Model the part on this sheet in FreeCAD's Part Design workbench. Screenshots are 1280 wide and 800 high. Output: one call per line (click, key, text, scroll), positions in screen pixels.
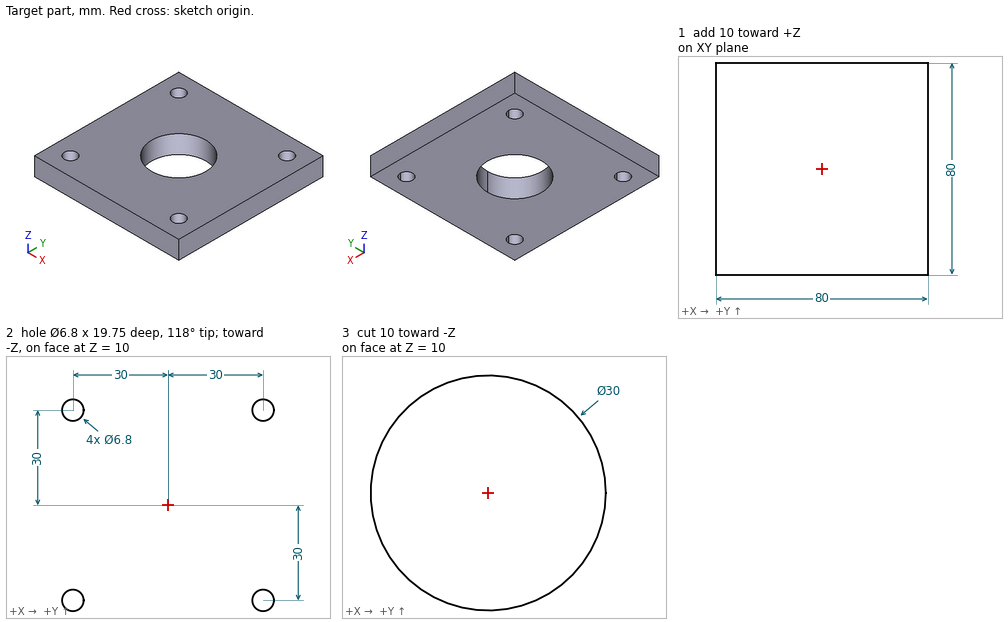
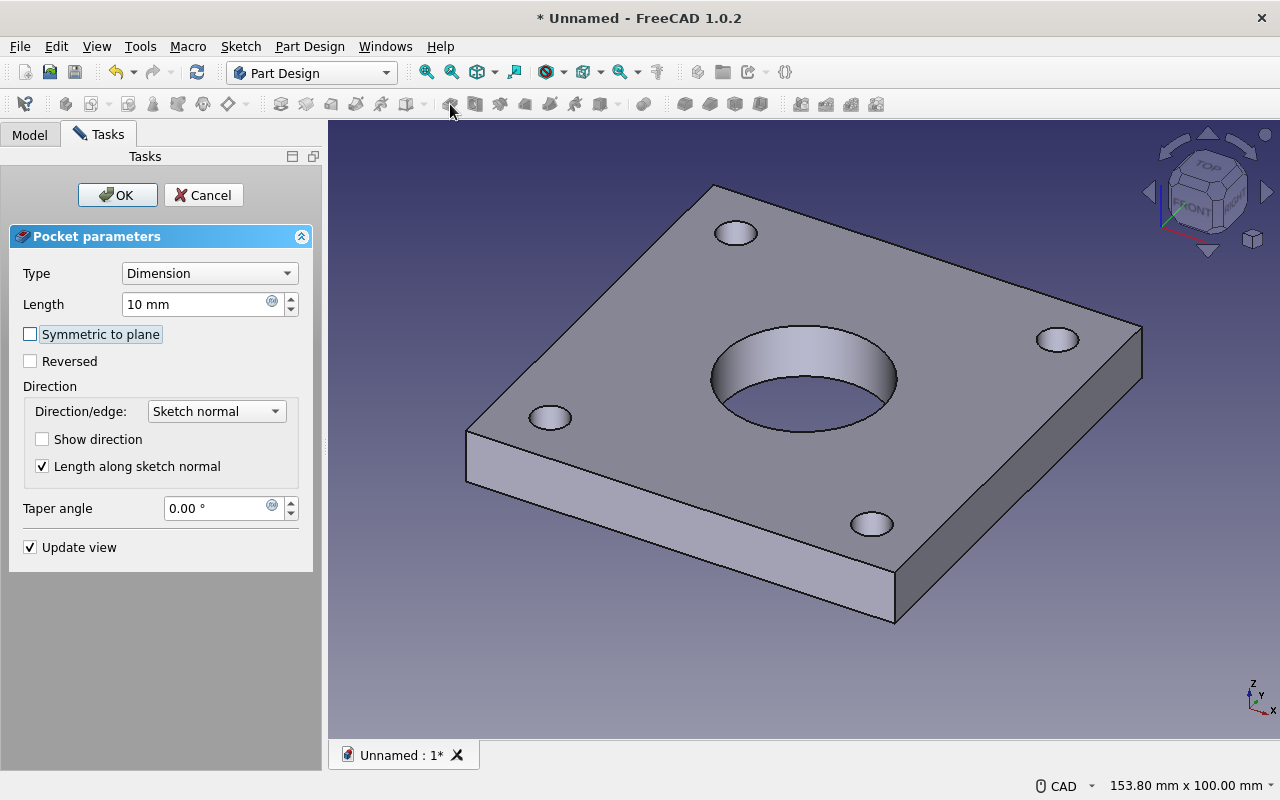
click(118, 195)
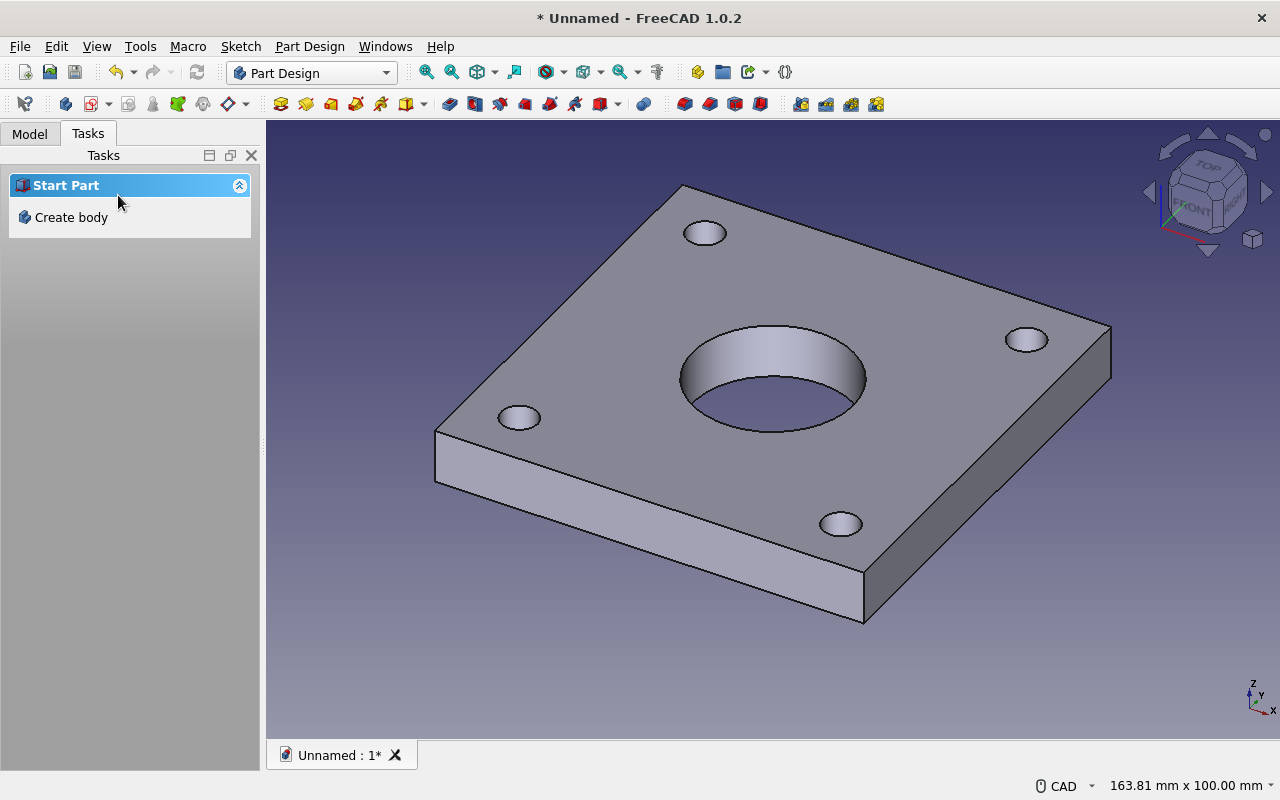
key(0)